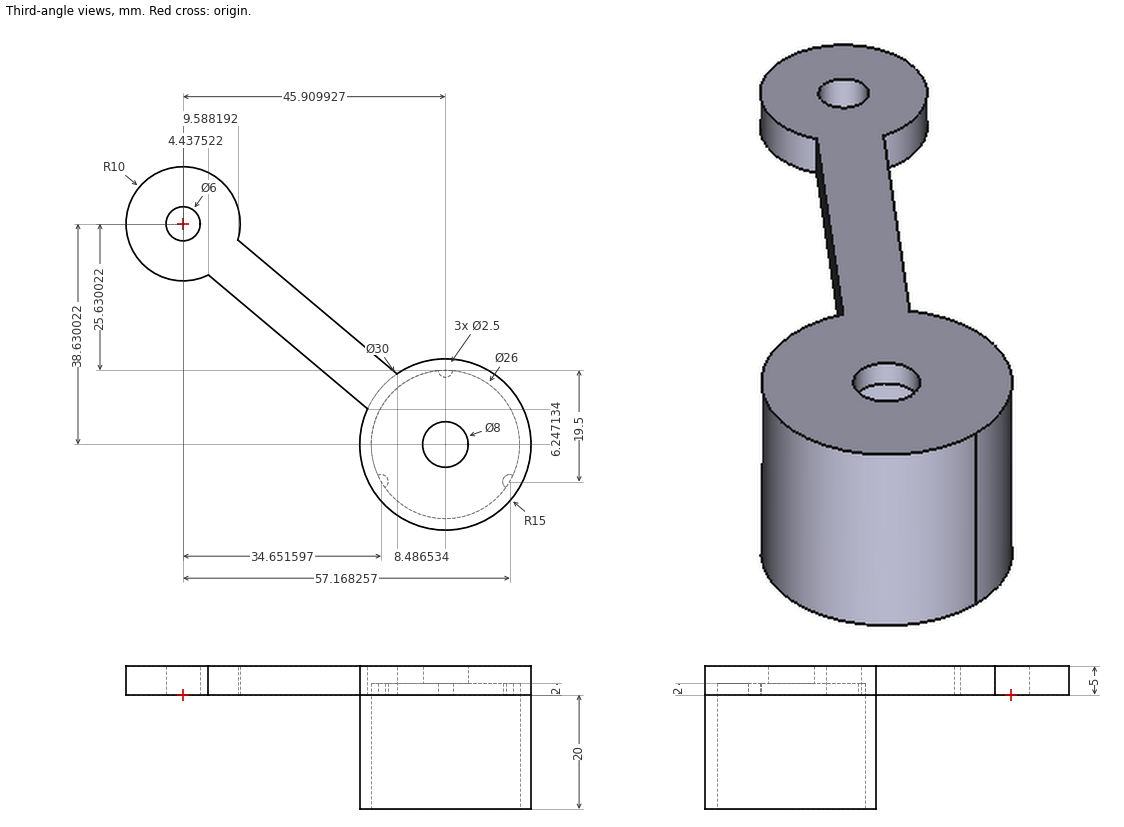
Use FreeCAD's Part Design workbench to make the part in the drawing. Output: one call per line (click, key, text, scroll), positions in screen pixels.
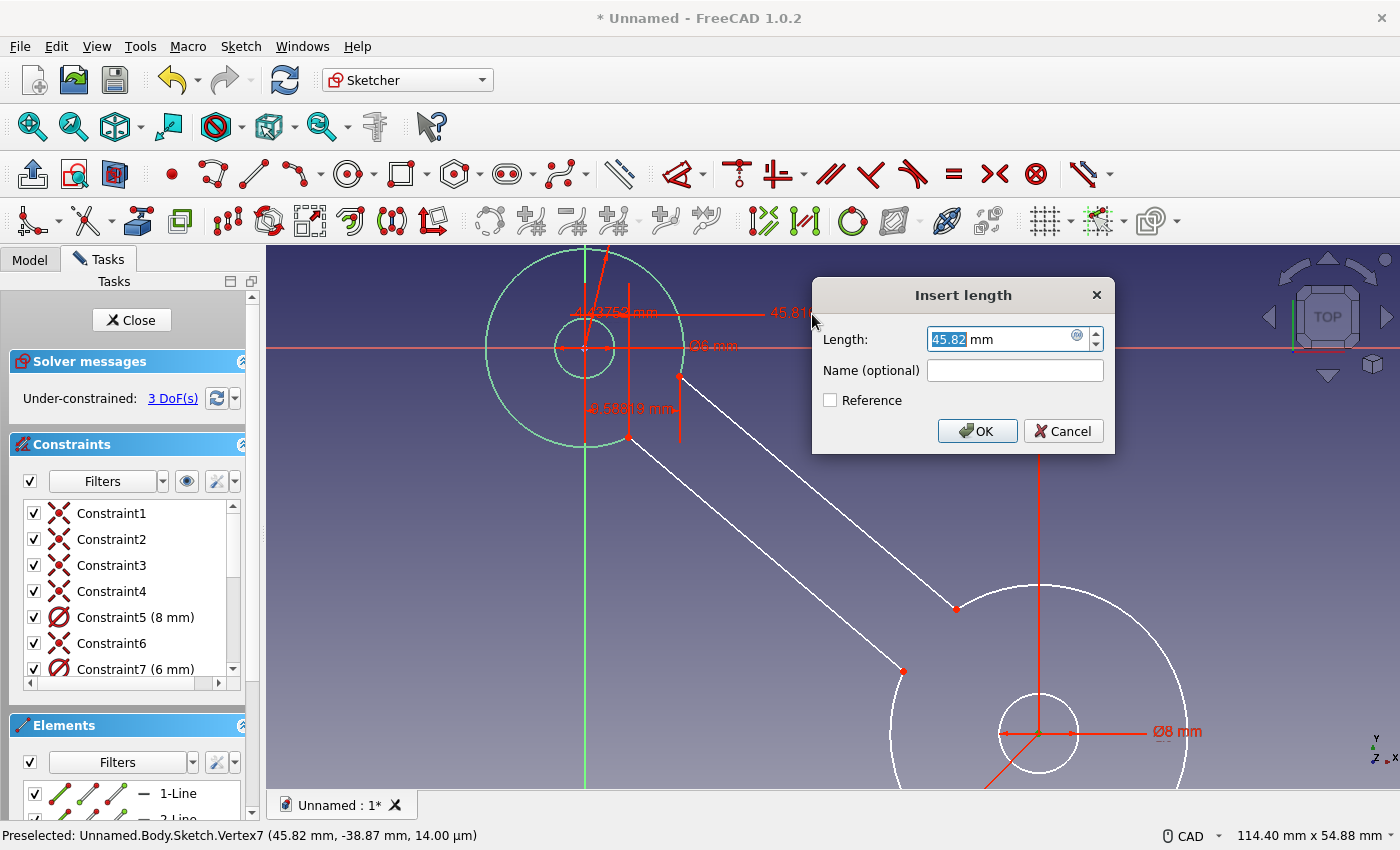
text(45.909927)
key(Return)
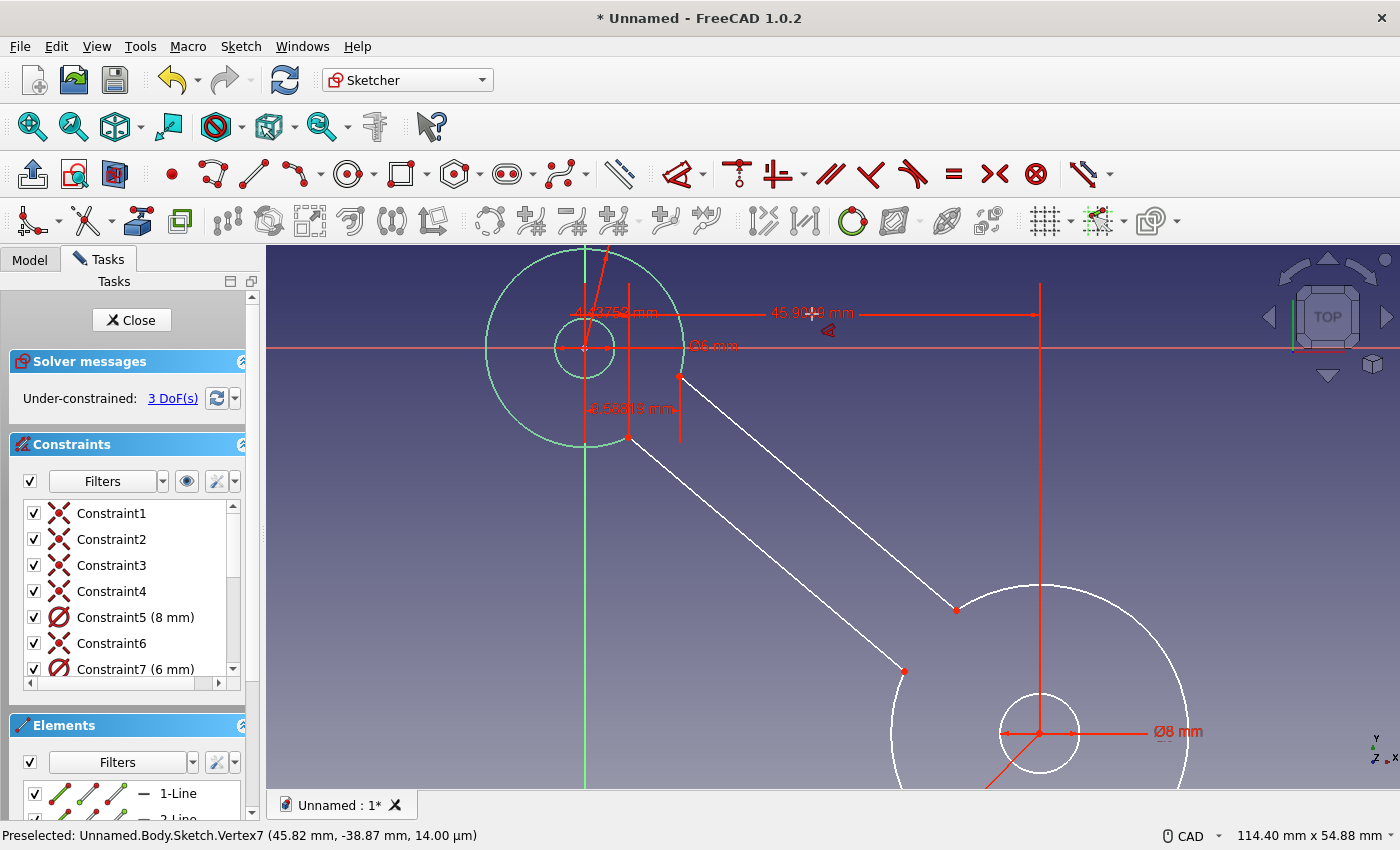
click(1040, 734)
click(551, 541)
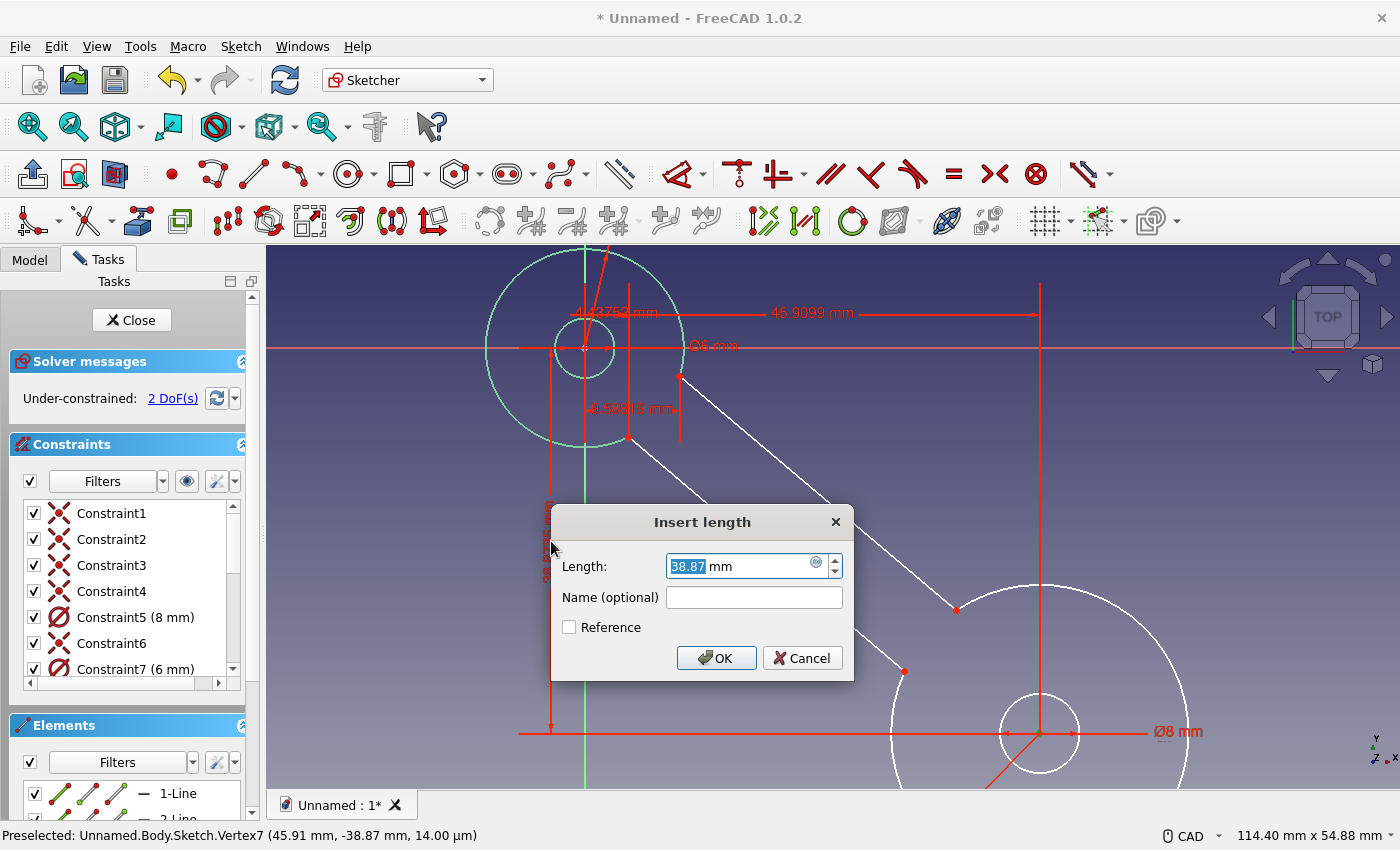
text(38.630022)
key(Return)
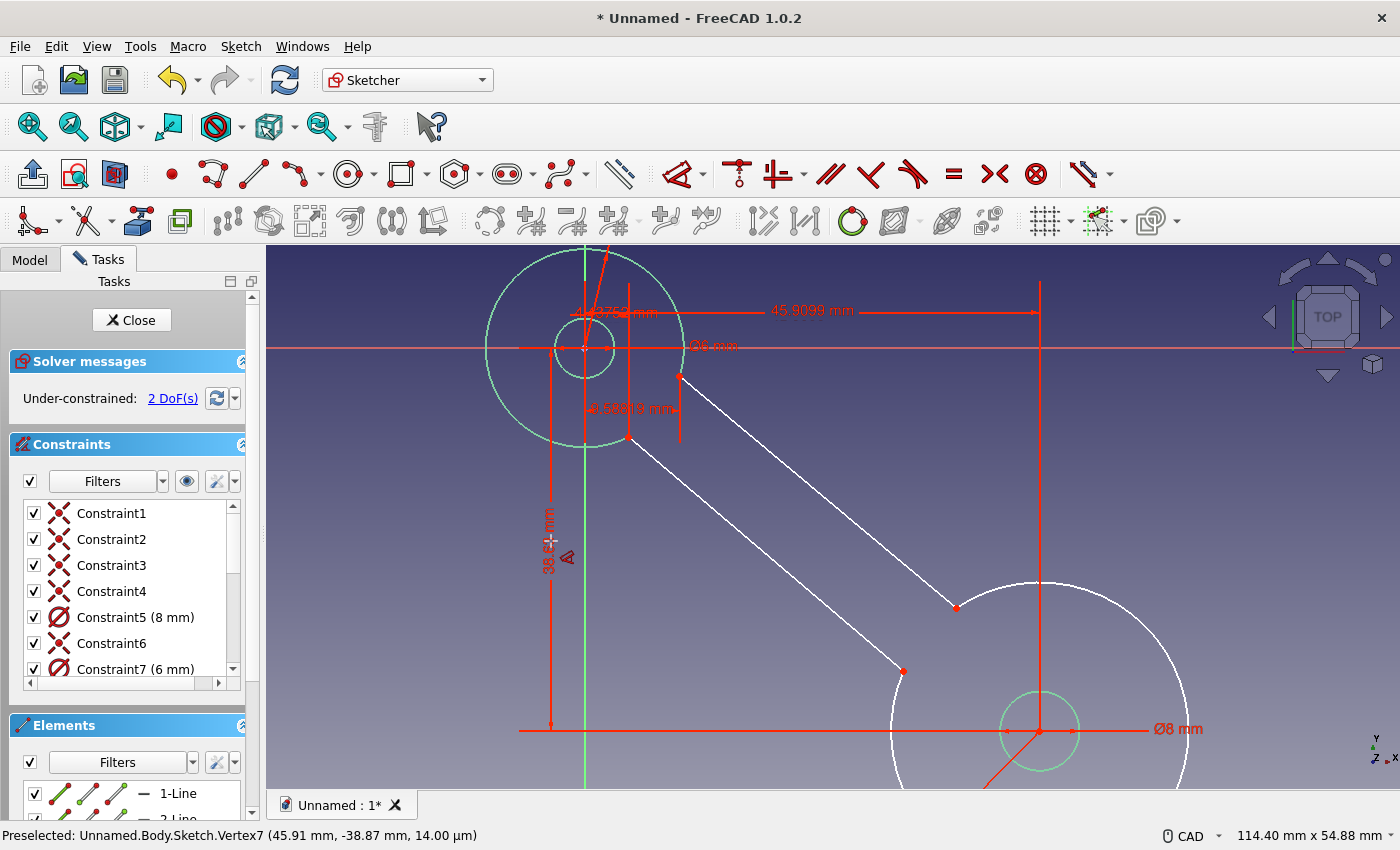
click(956, 608)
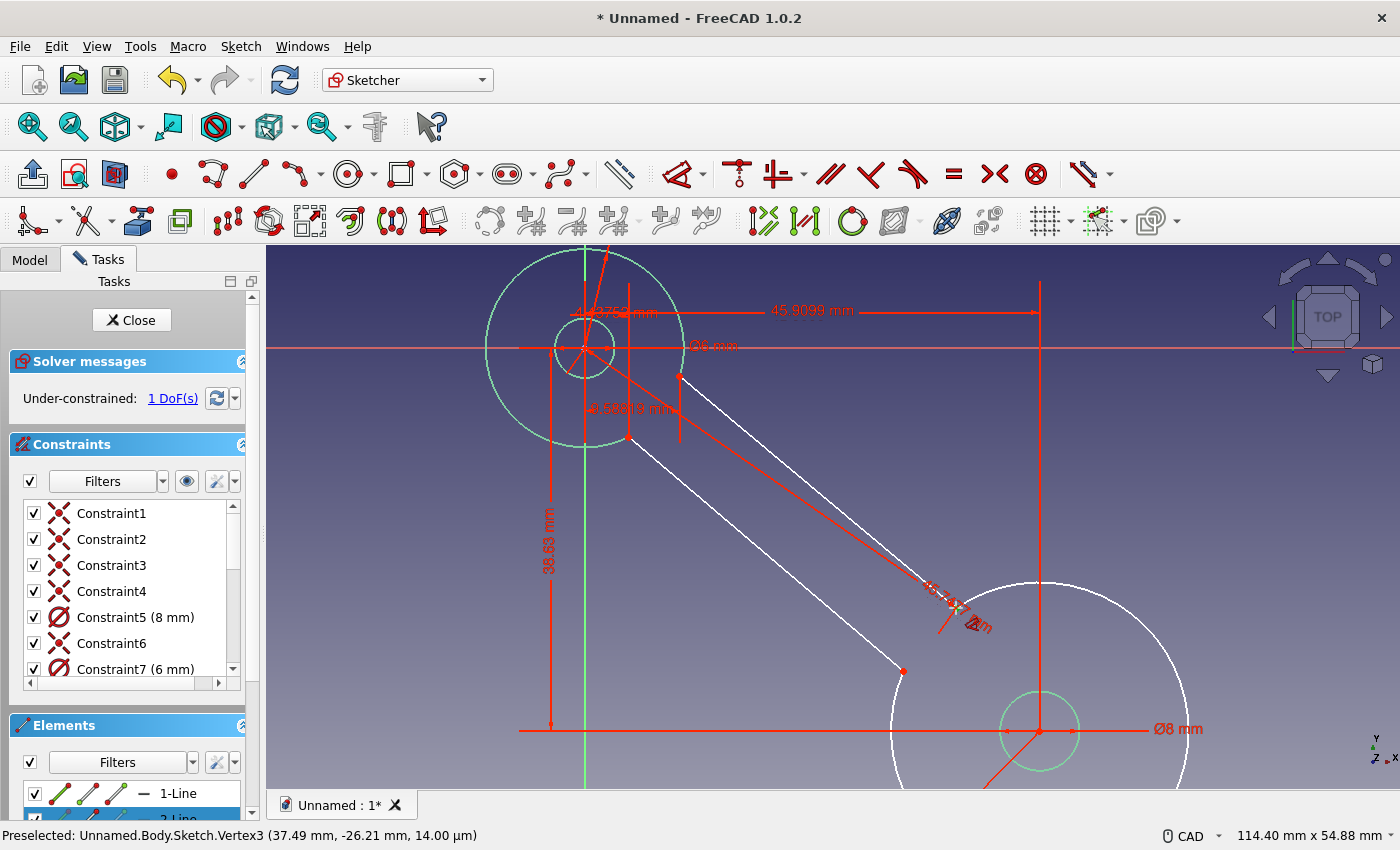
click(1040, 731)
click(998, 574)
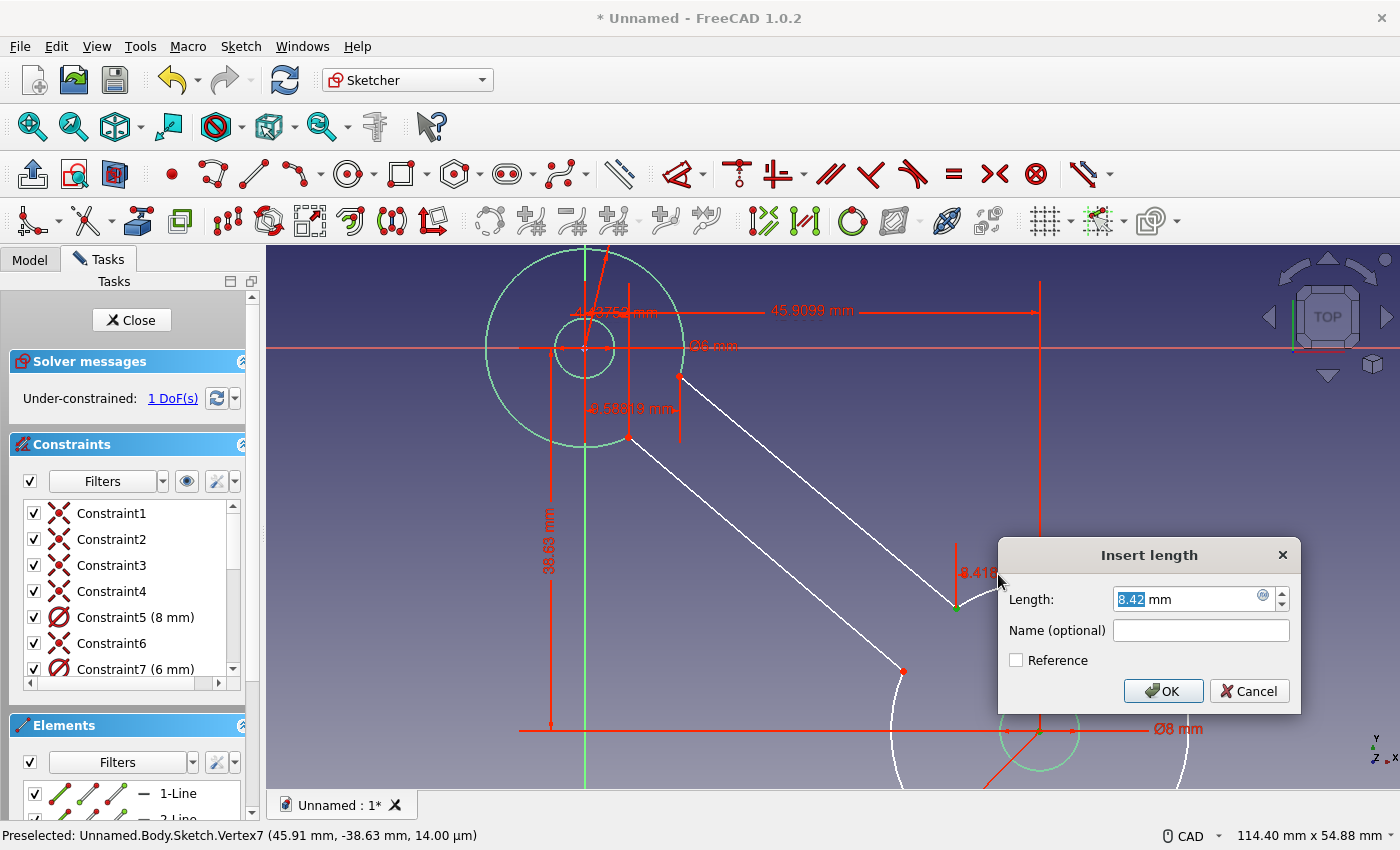
text(8.486534)
key(Return)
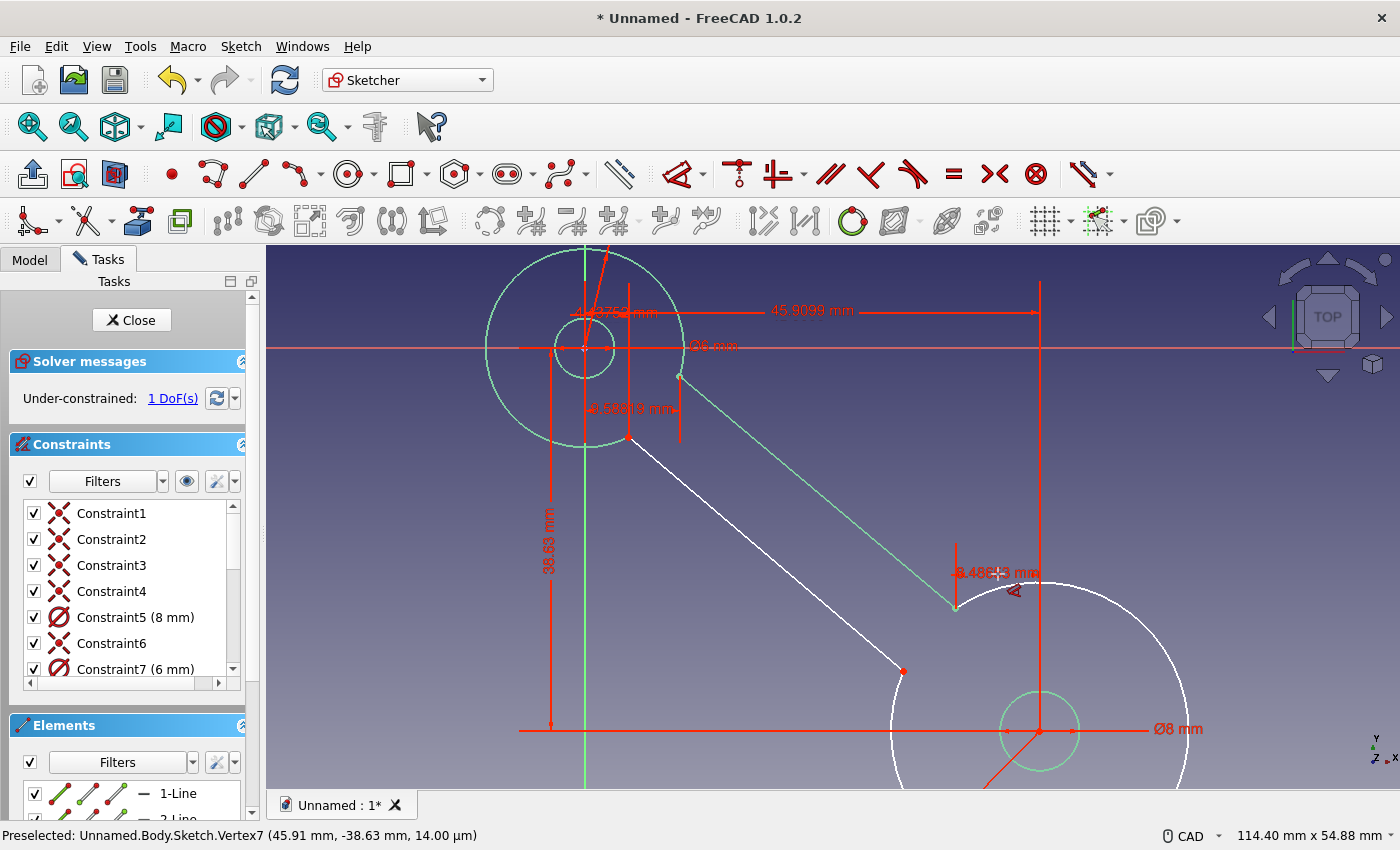
click(904, 671)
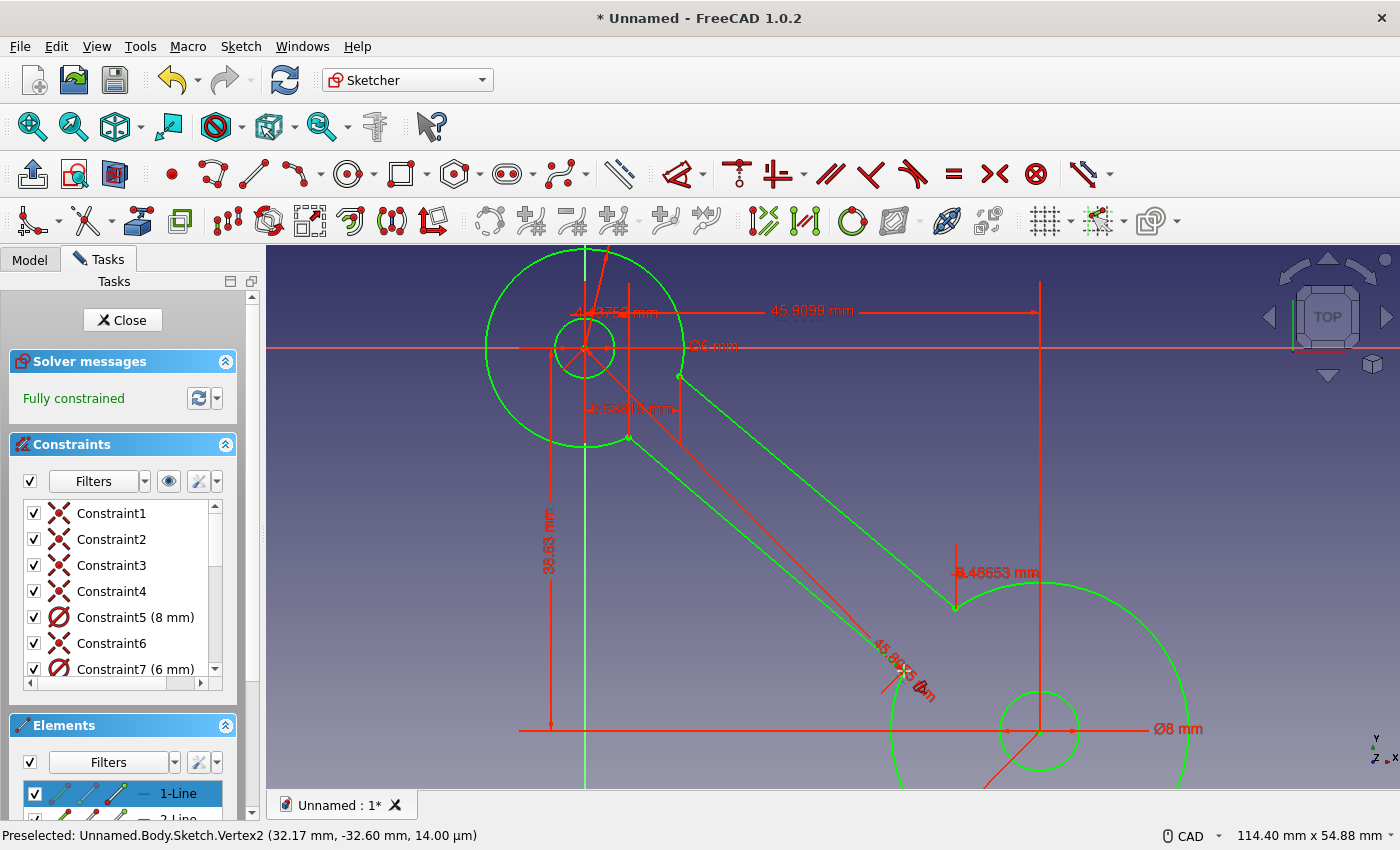
click(1040, 731)
click(1074, 688)